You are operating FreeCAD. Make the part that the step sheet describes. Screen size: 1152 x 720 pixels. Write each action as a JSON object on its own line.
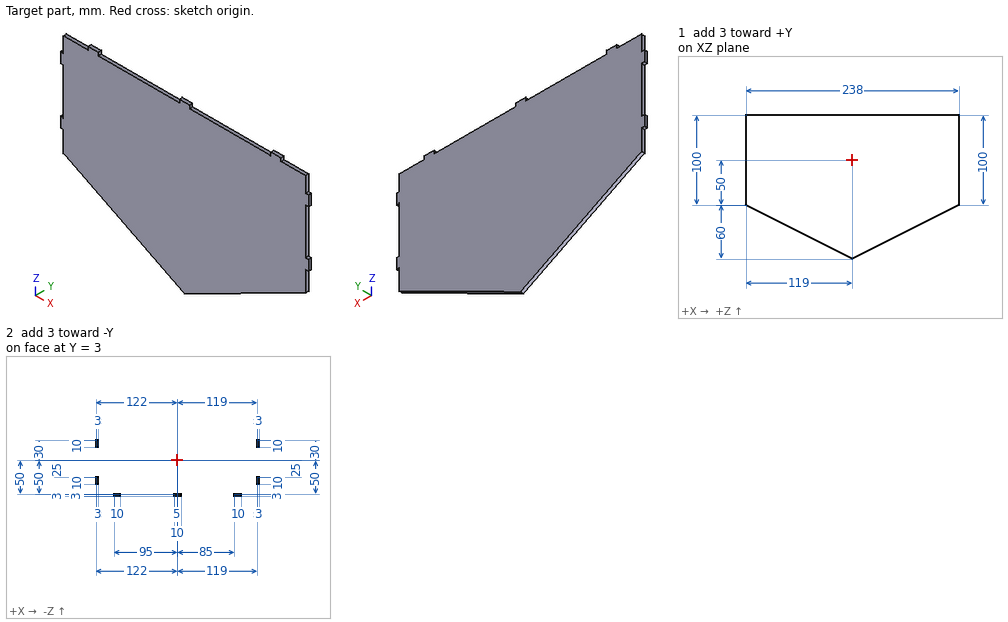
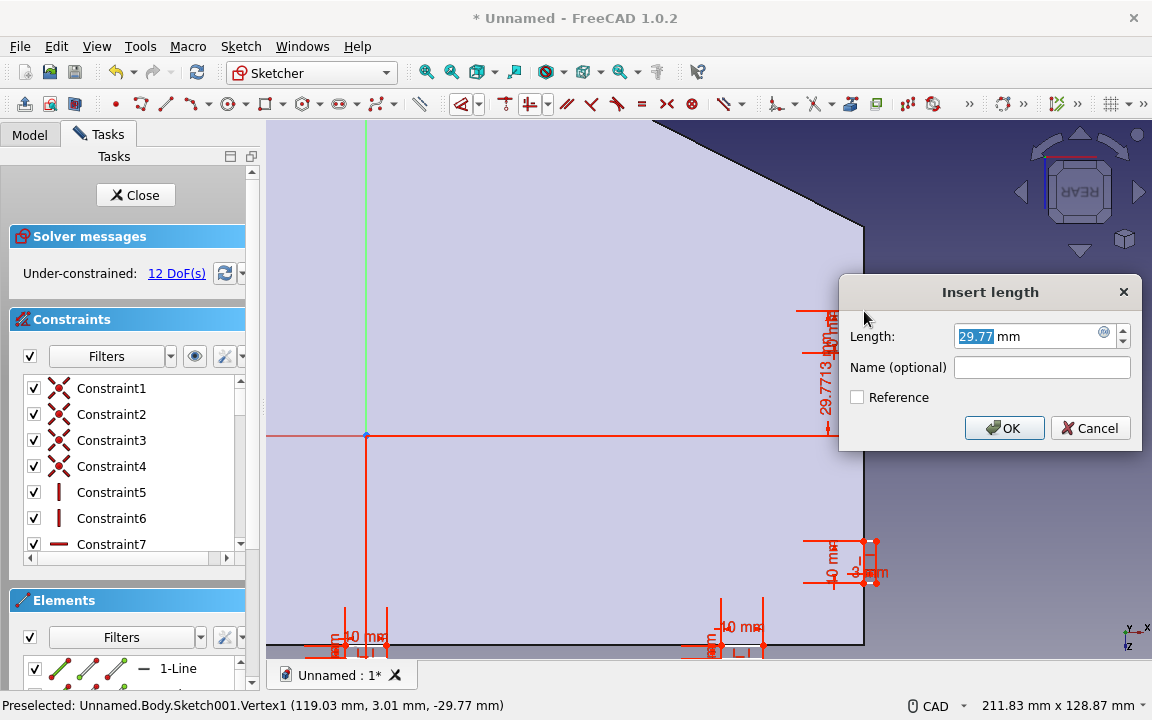
{"action": "type", "text": "30"}
{"action": "key", "text": "Return"}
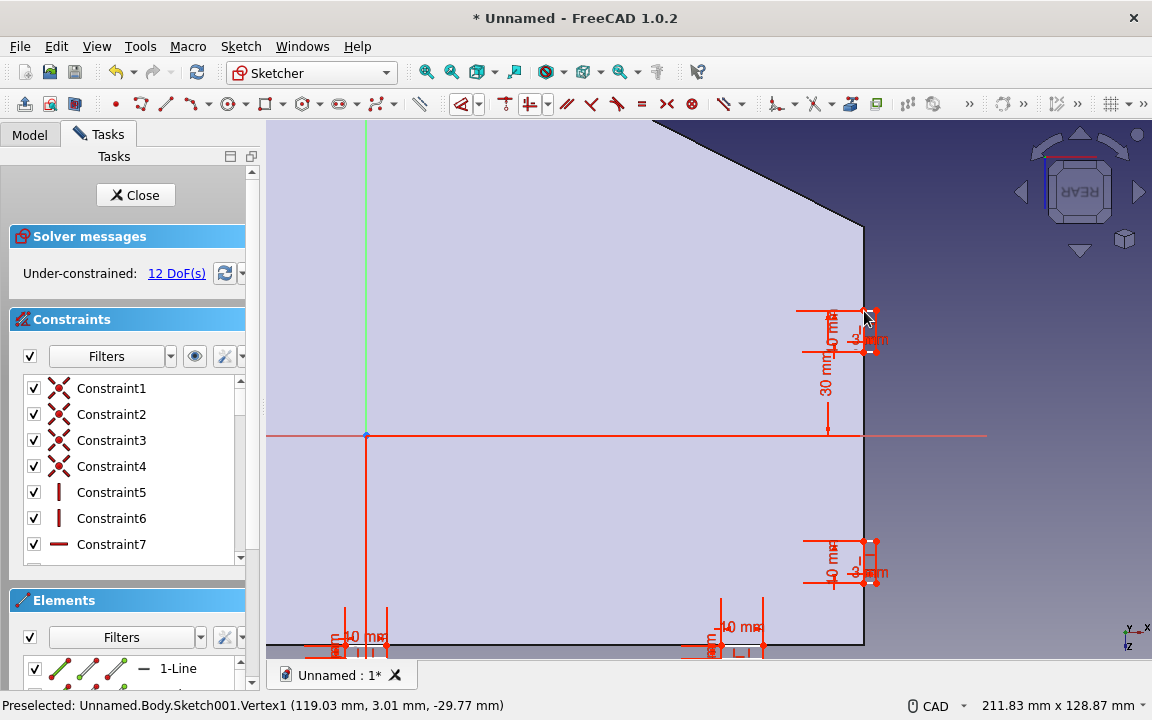
{"action": "left_click", "coordinate": [864, 541]}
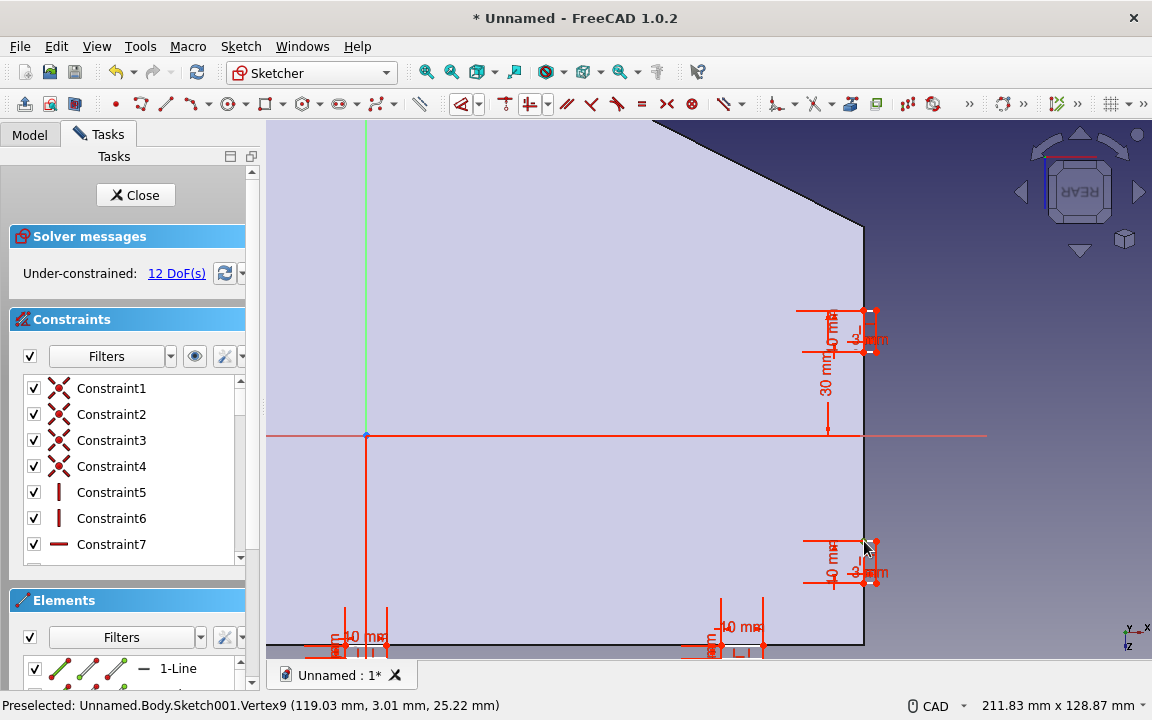
{"action": "key", "text": "i"}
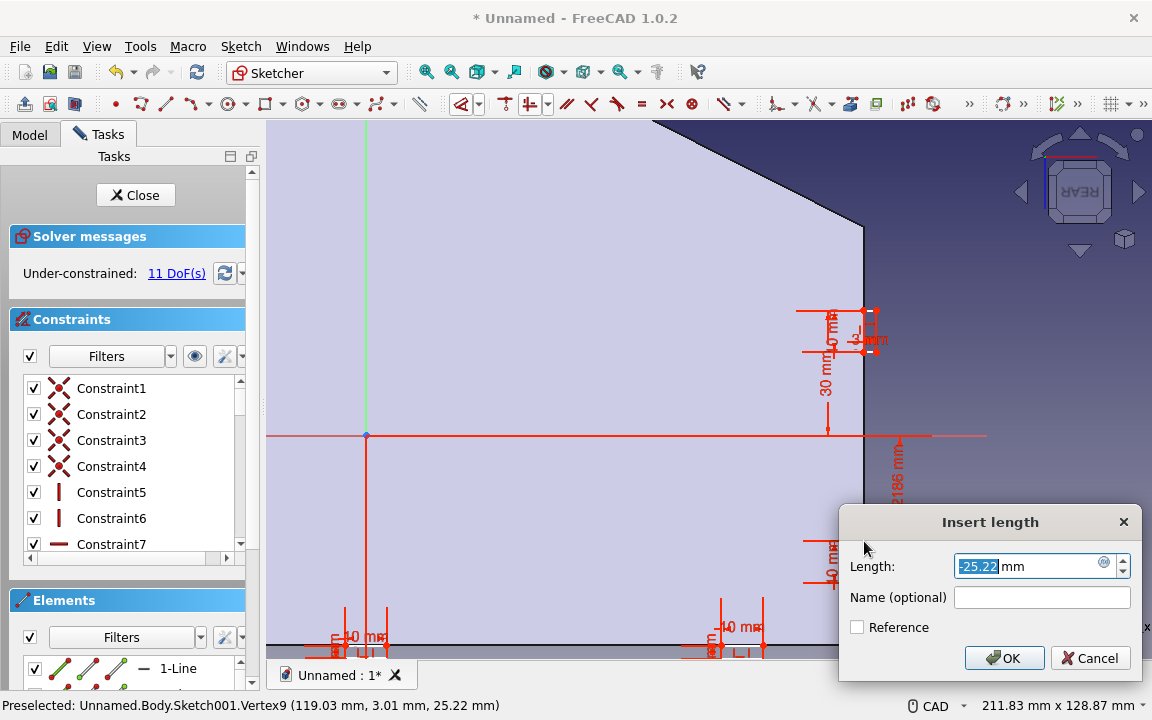
{"action": "type", "text": "-25"}
{"action": "key", "text": "Return"}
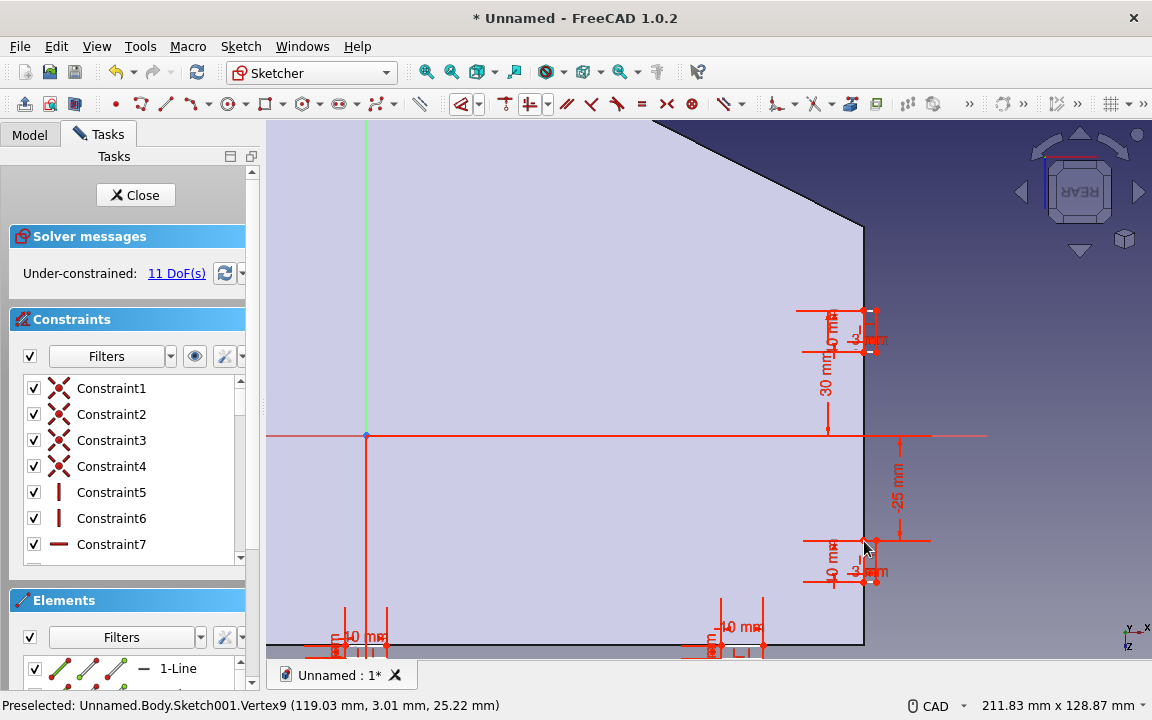
{"action": "scroll", "coordinate": [864, 312], "scroll_direction": "down", "scroll_amount": 4}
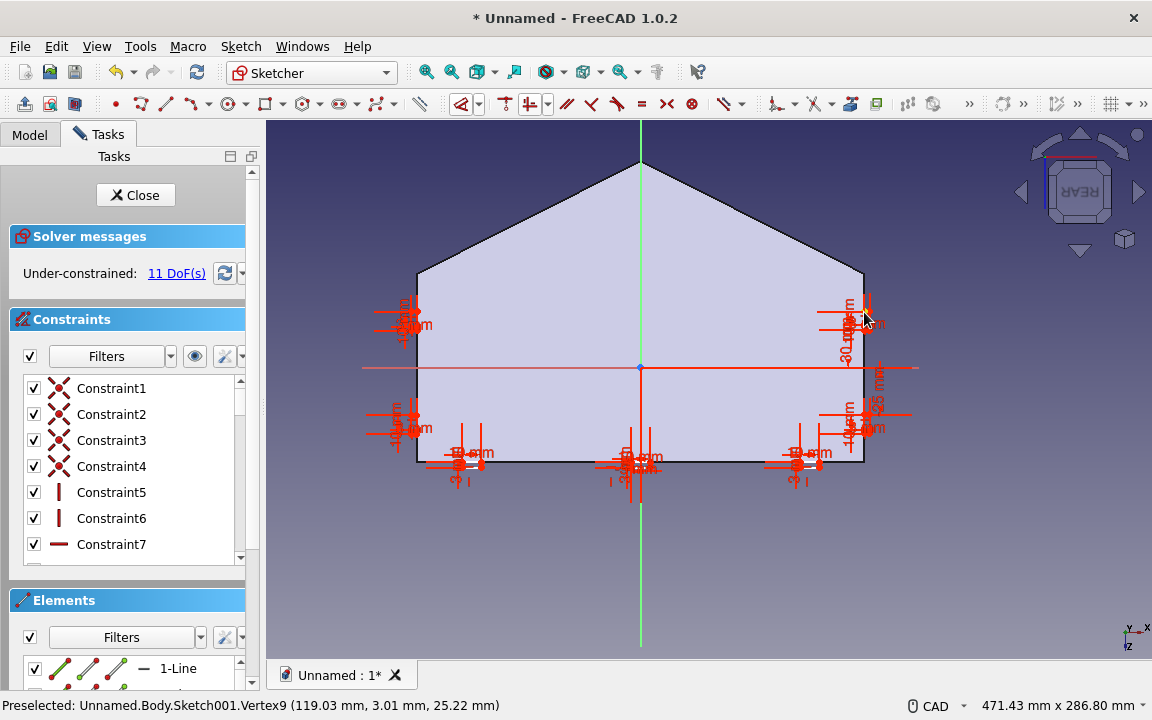
{"action": "scroll", "coordinate": [411, 415], "scroll_direction": "up", "scroll_amount": 4}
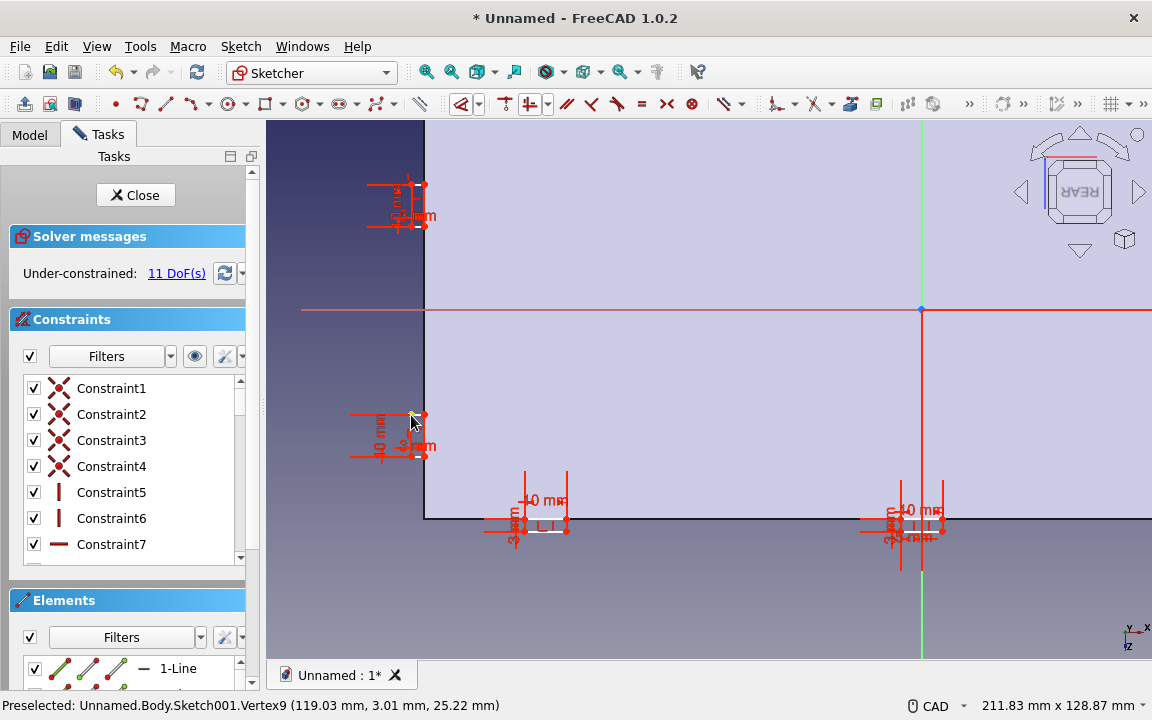
{"action": "left_click", "coordinate": [411, 415]}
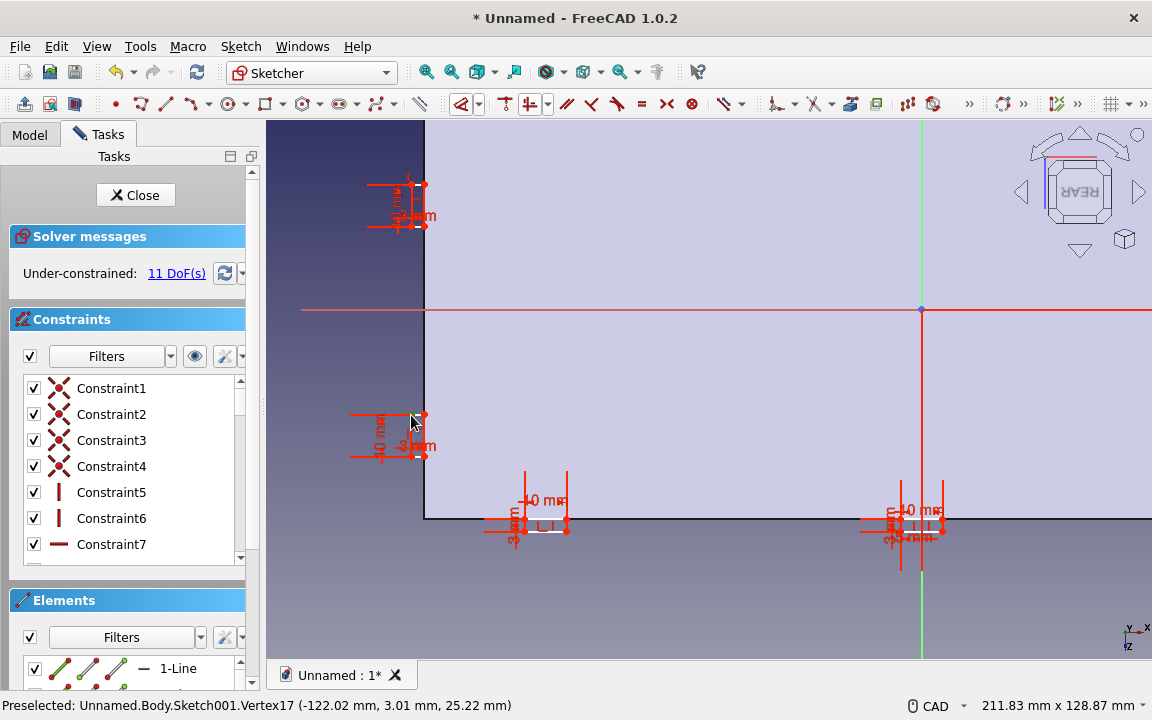
{"action": "key", "text": "i"}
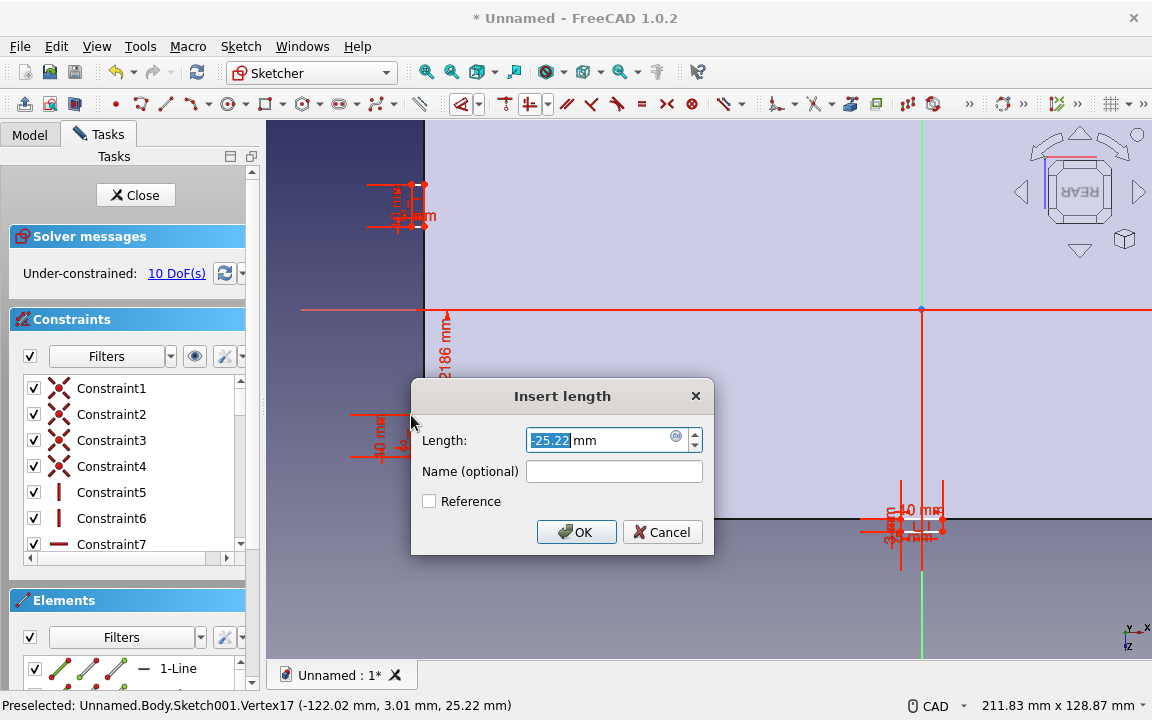
{"action": "type", "text": "-25"}
{"action": "key", "text": "Return"}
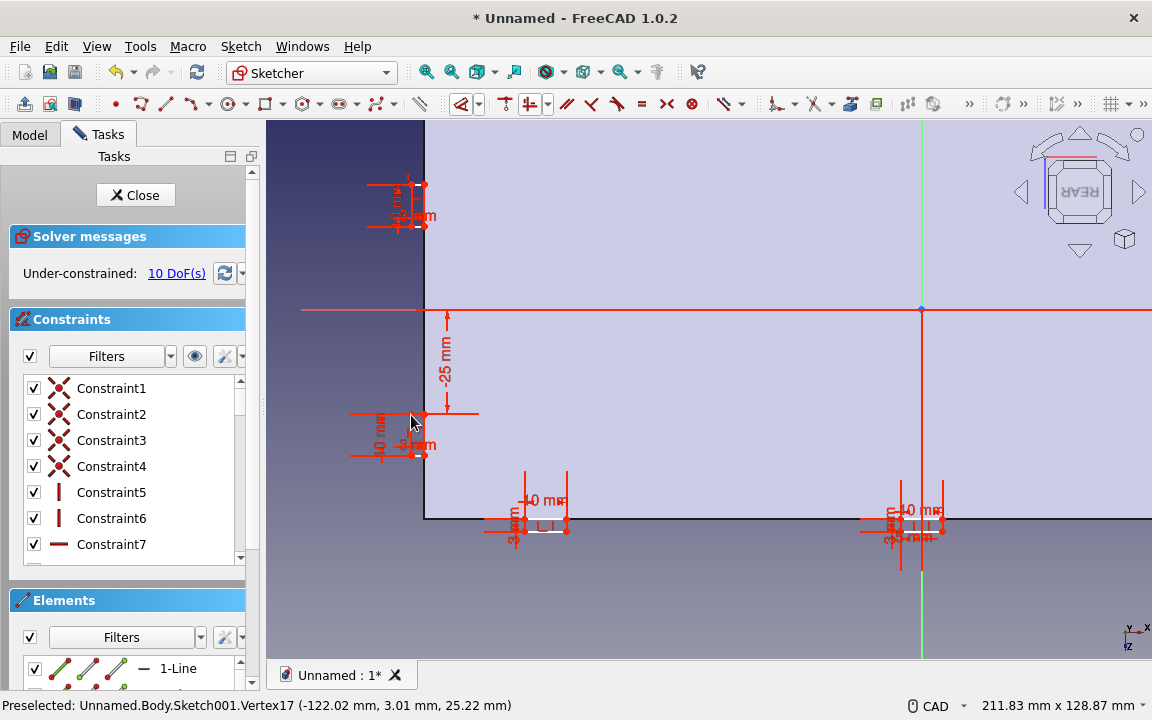
{"action": "left_click", "coordinate": [412, 185]}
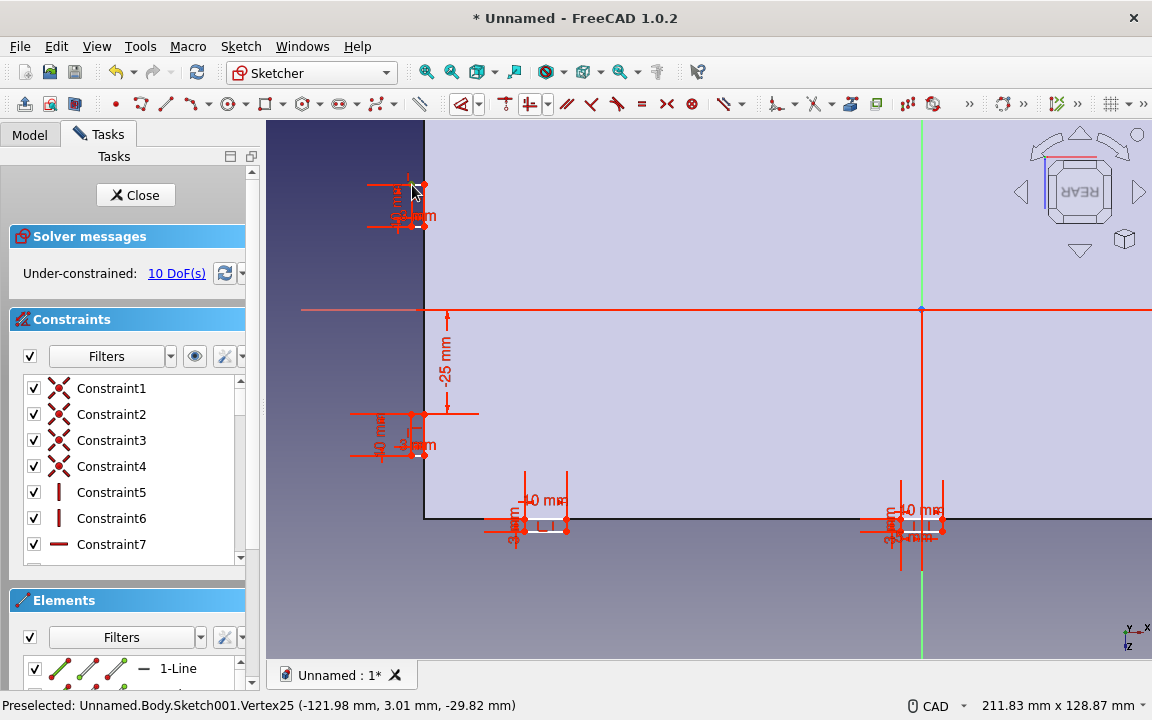
{"action": "key", "text": "i"}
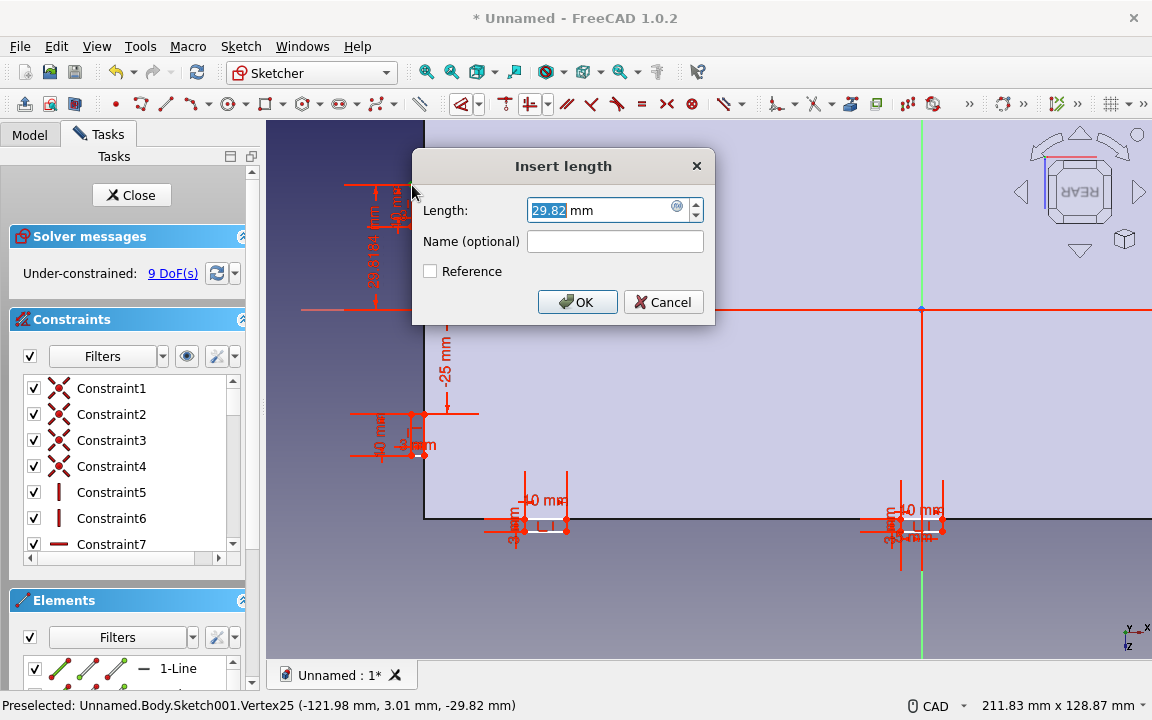
{"action": "type", "text": "30"}
{"action": "key", "text": "Return"}